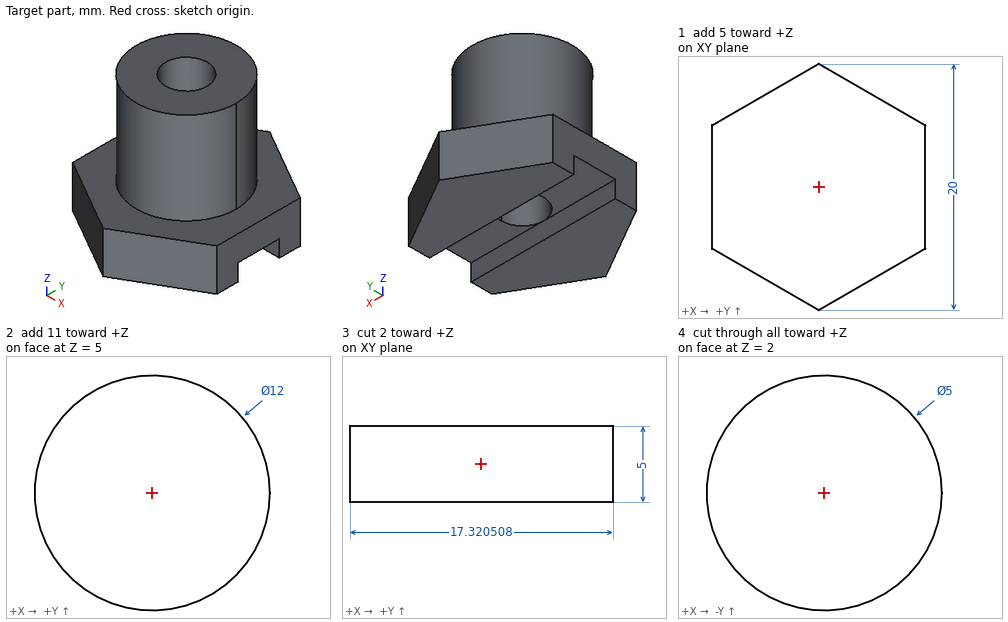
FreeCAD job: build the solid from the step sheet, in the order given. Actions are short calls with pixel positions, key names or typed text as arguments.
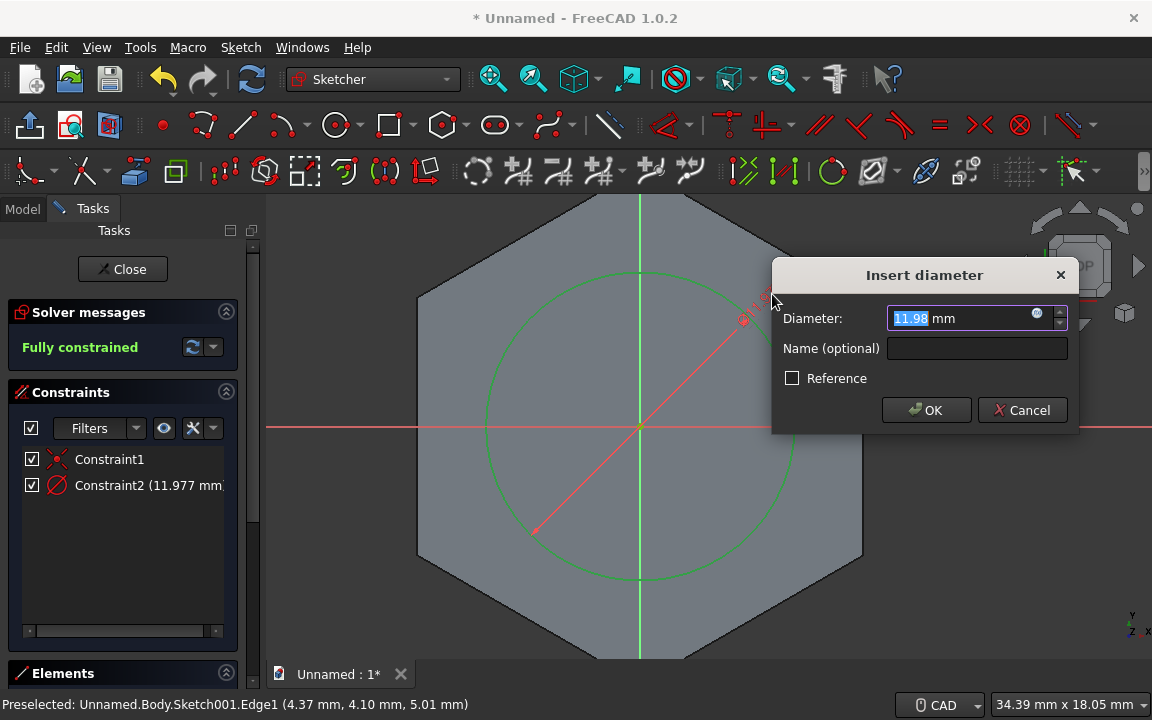
text(12)
key(Return)
key(Escape)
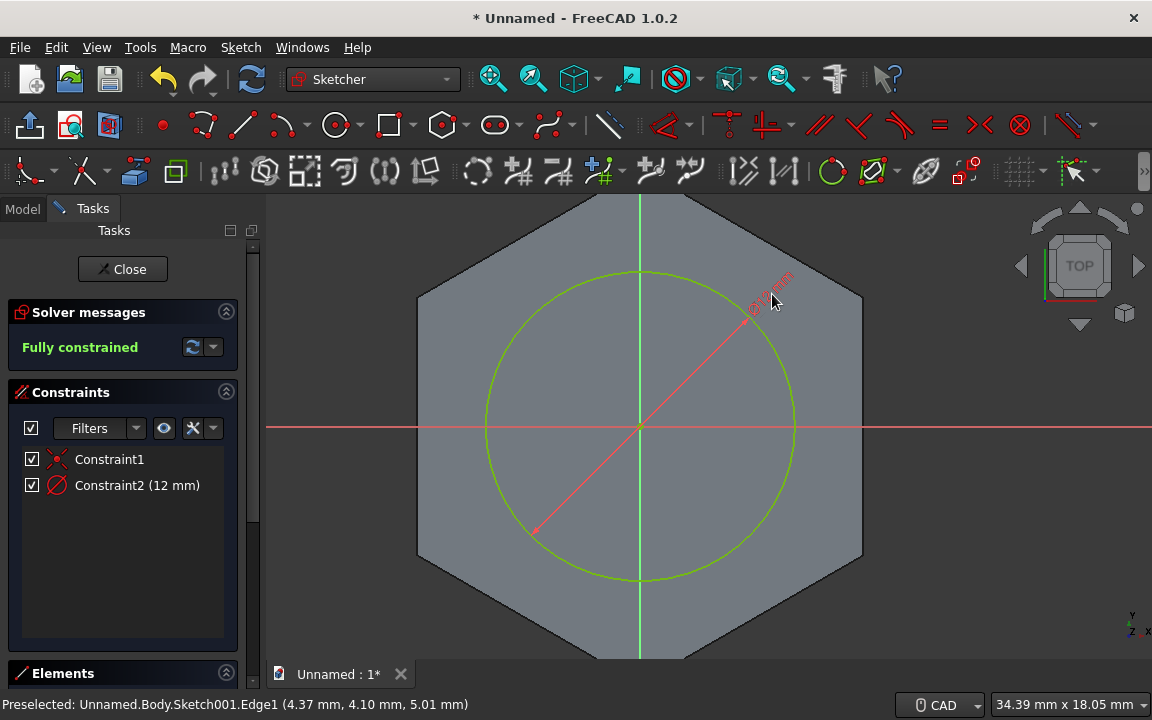
click(123, 269)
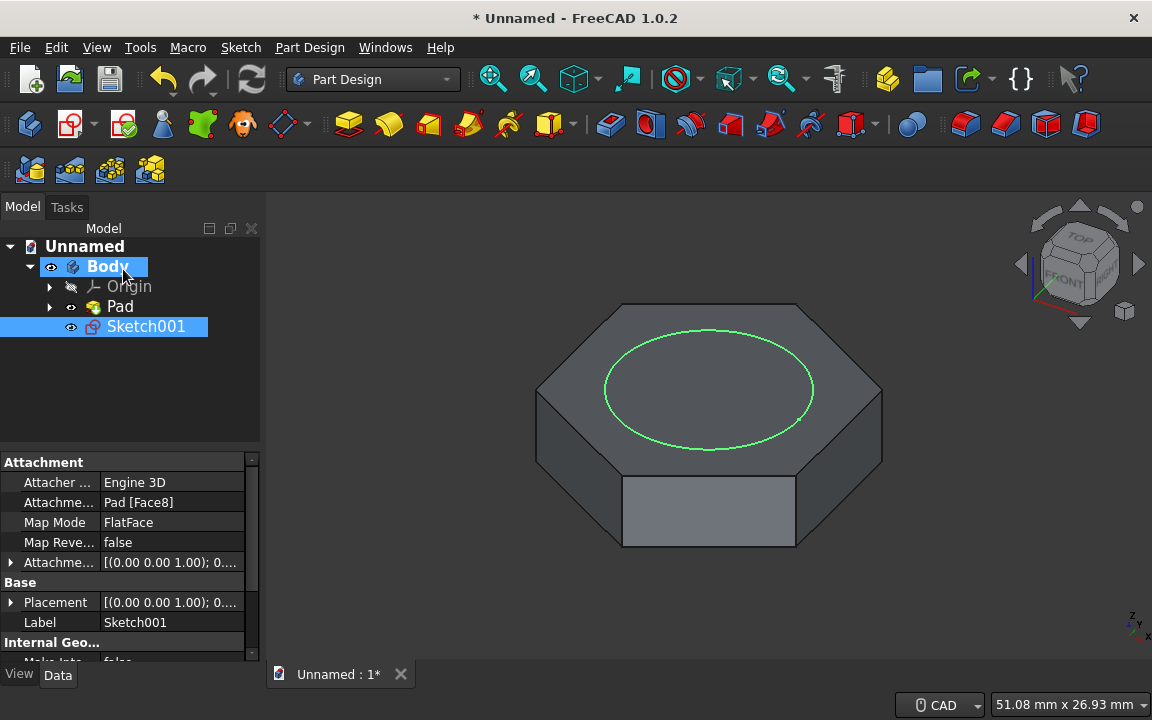
click(350, 124)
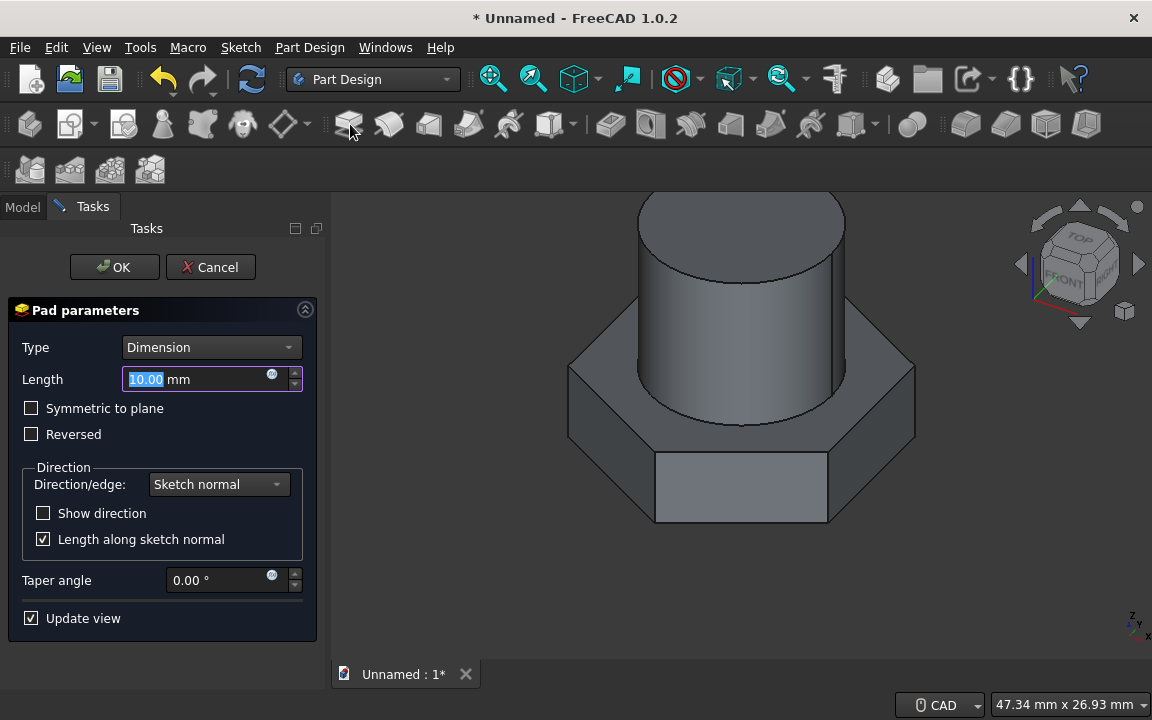
text(11)
key(Tab)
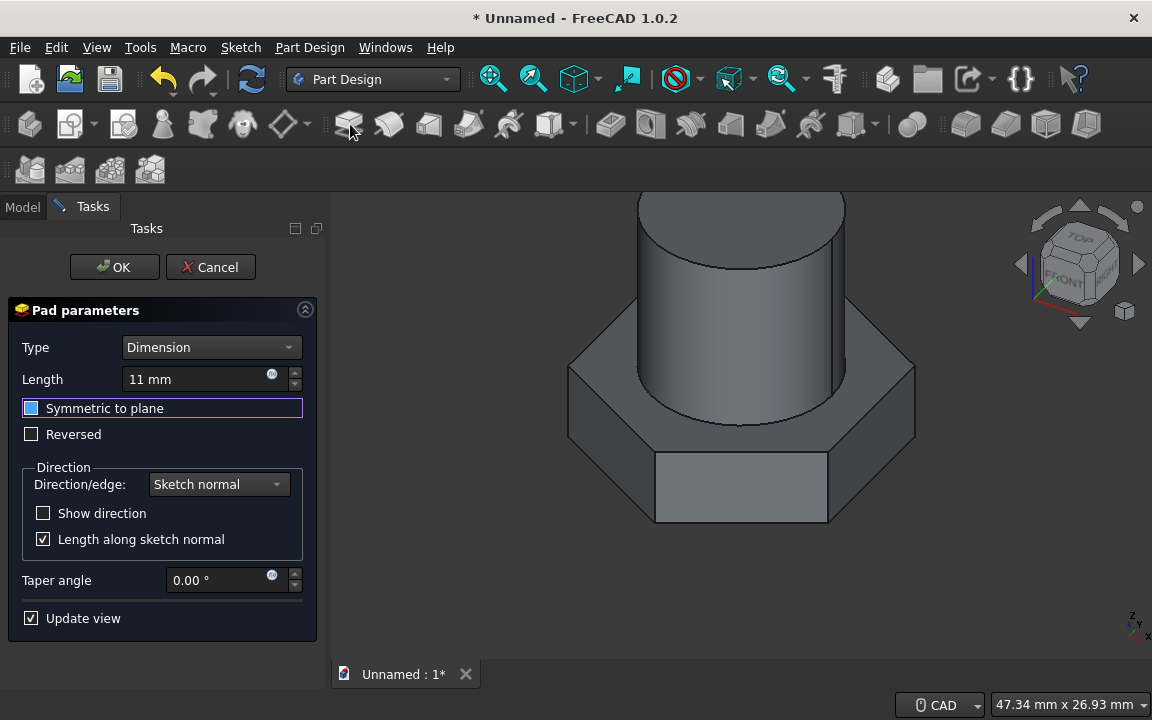
click(115, 267)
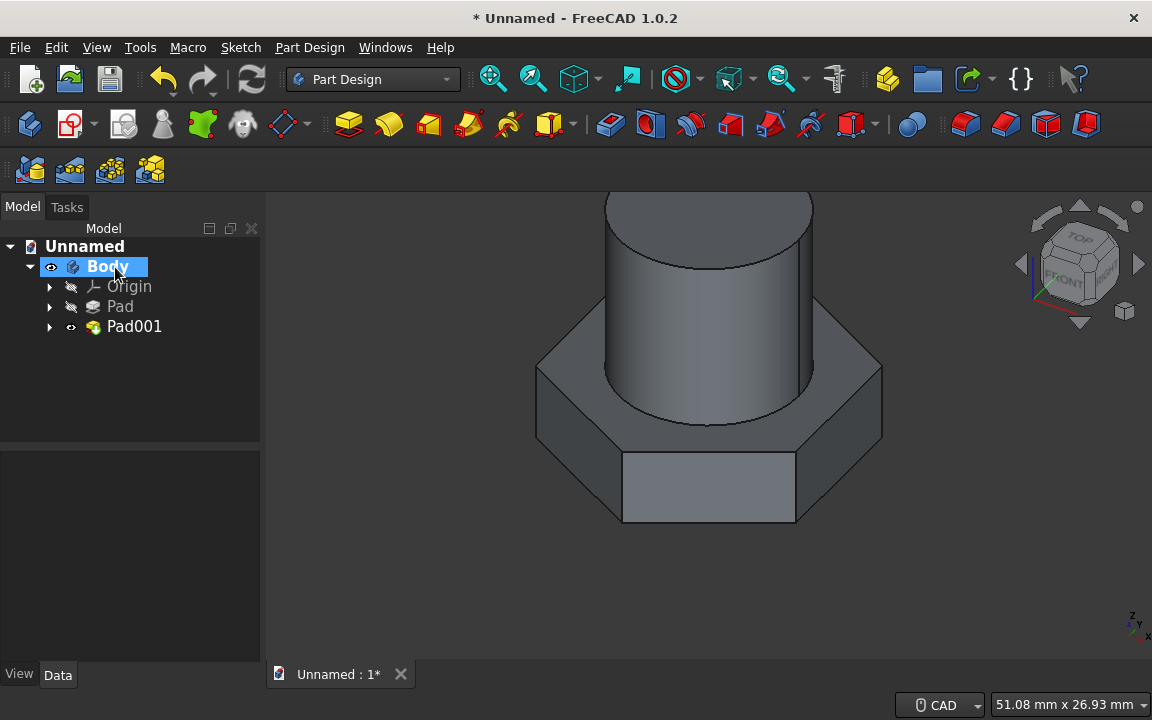
key(v)
key(f)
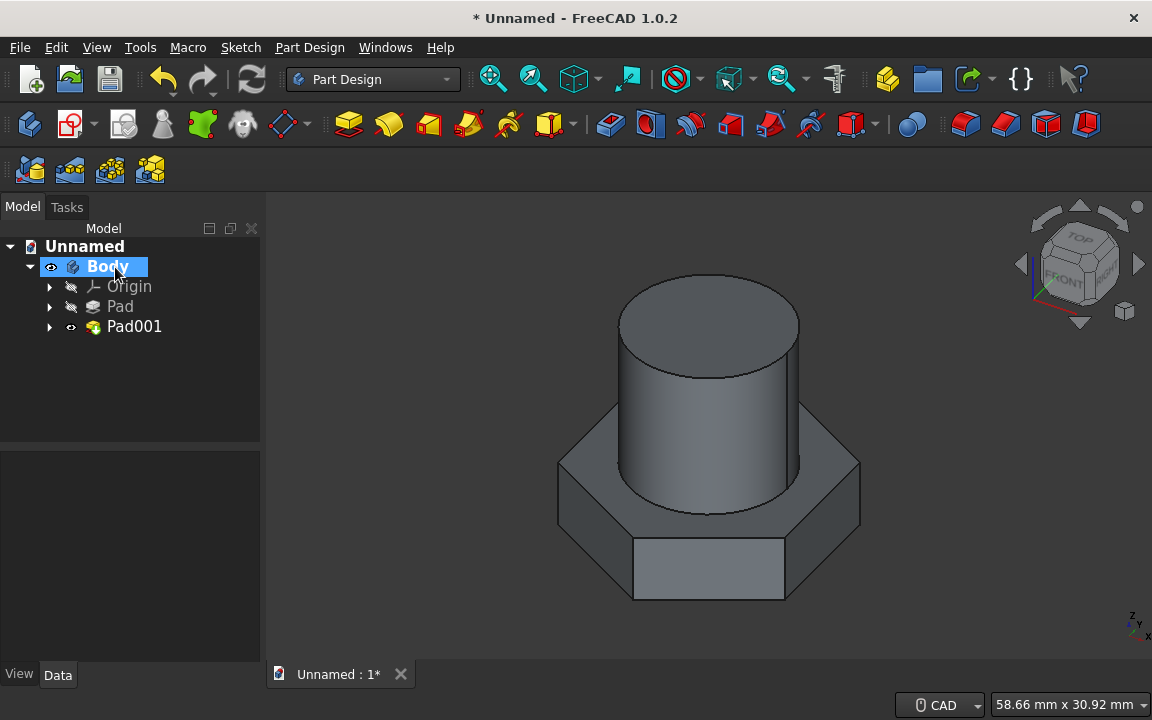
click(70, 124)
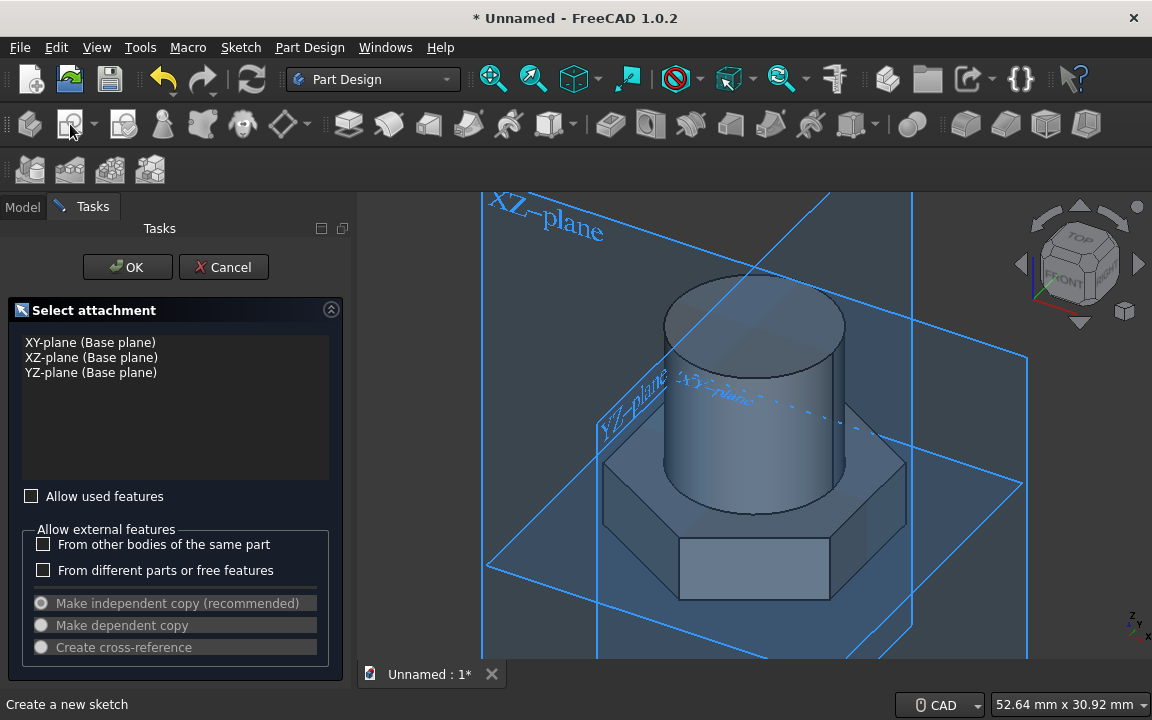
click(82, 342)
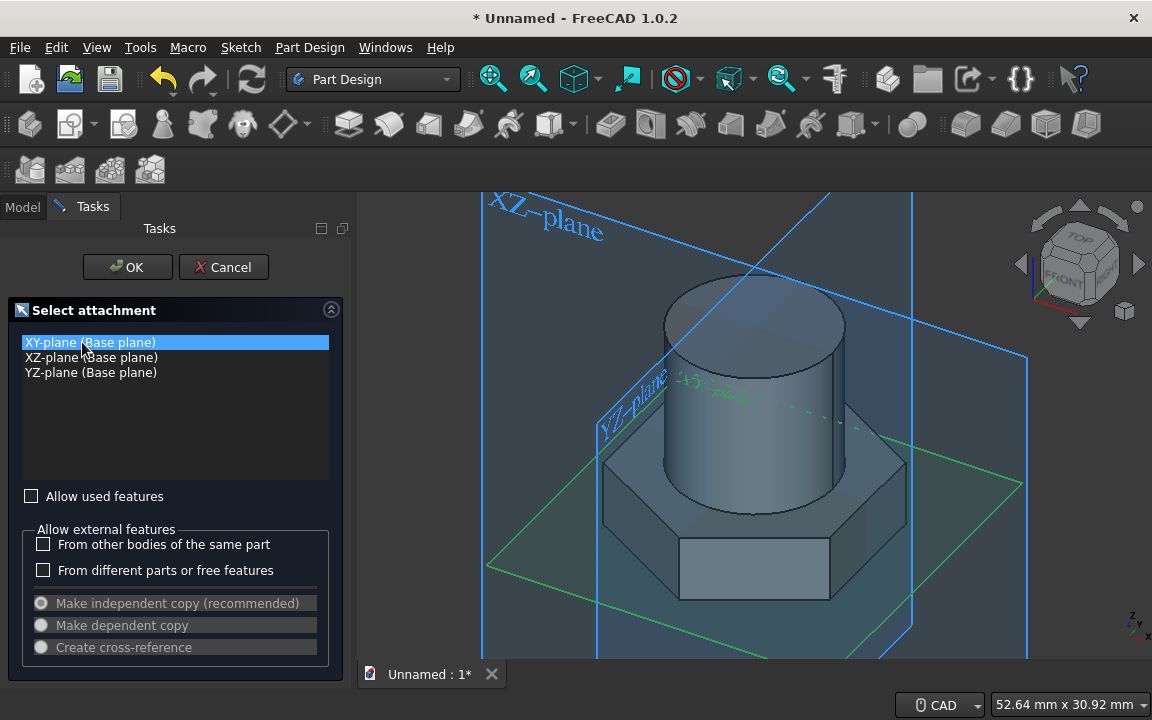
click(128, 267)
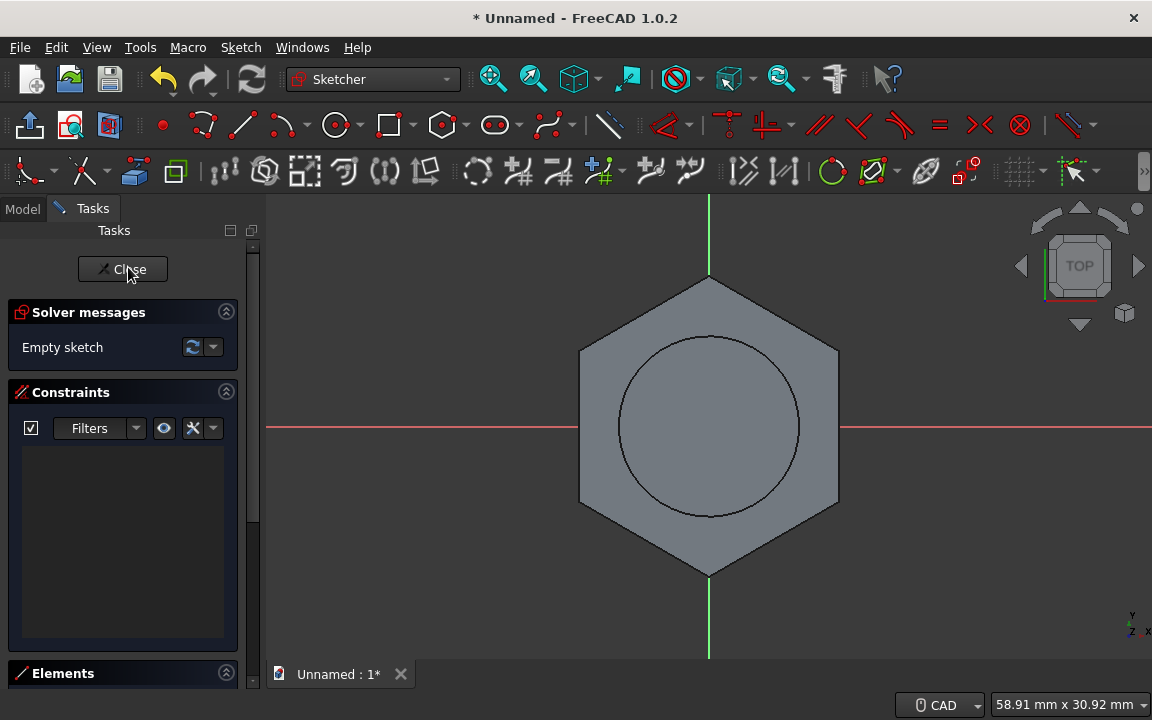
key(q)
key(s)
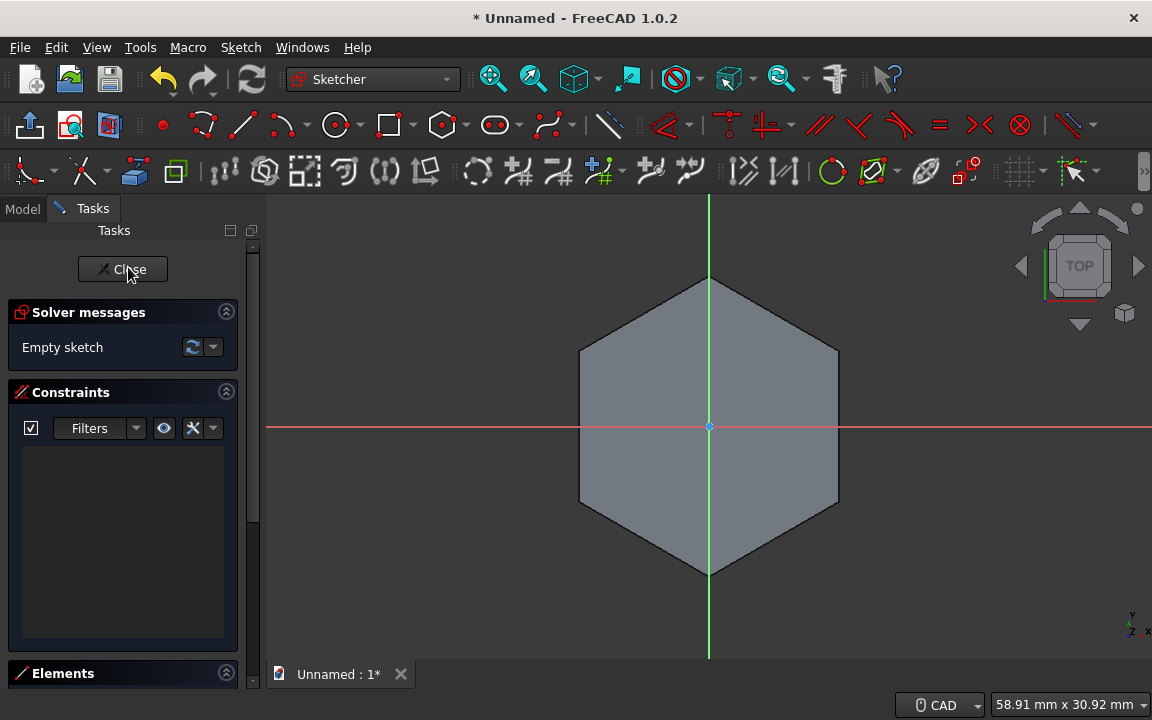
scroll(792, 426, up, 3)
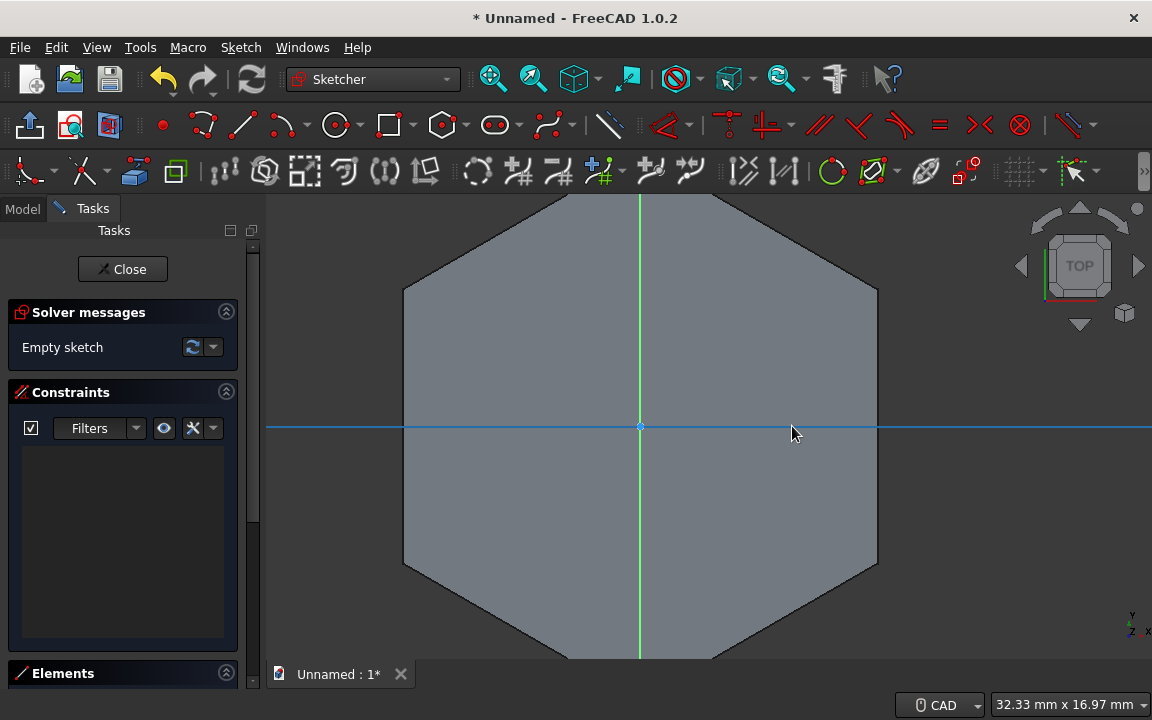
key(g)
key(v)